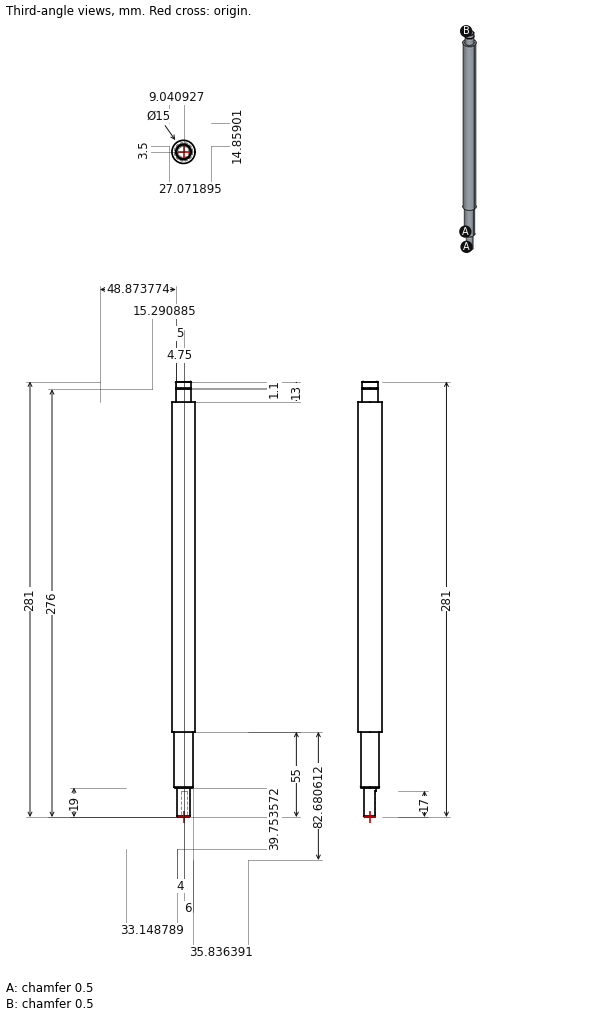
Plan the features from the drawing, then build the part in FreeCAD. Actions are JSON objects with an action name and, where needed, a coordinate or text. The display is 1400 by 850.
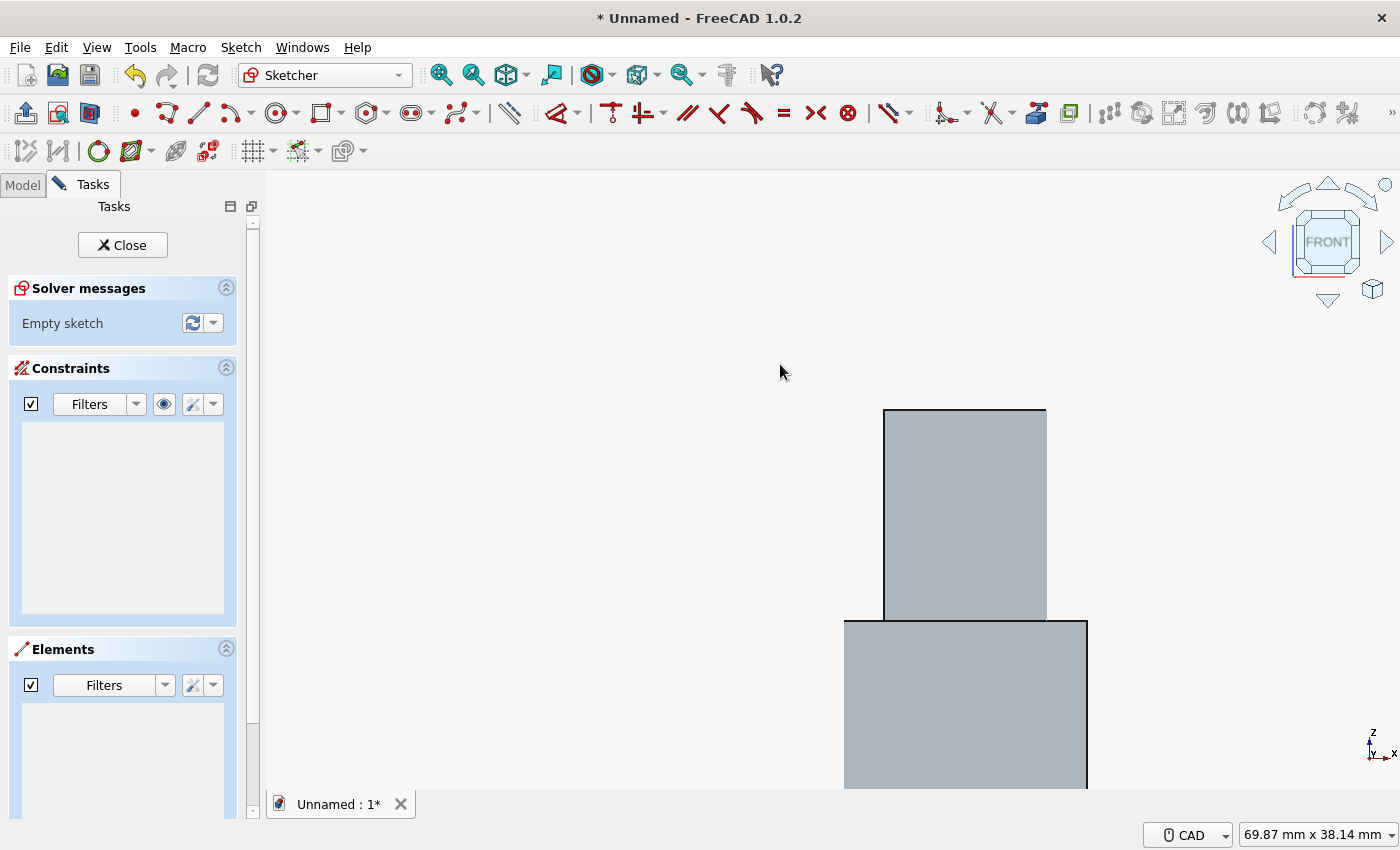
{"action": "scroll", "coordinate": [764, 484], "scroll_direction": "up", "scroll_amount": 5}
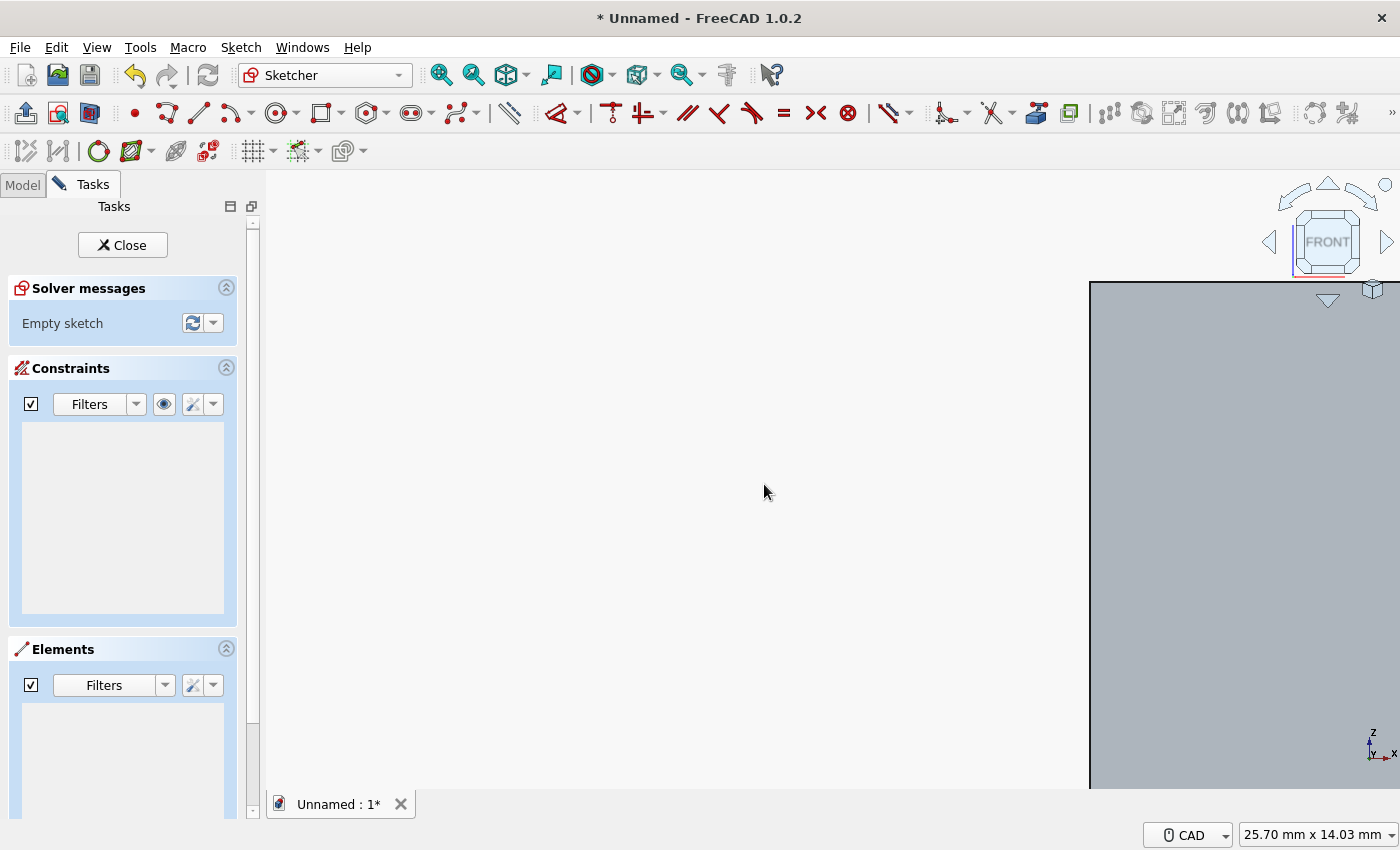
{"action": "left_click", "coordinate": [322, 114]}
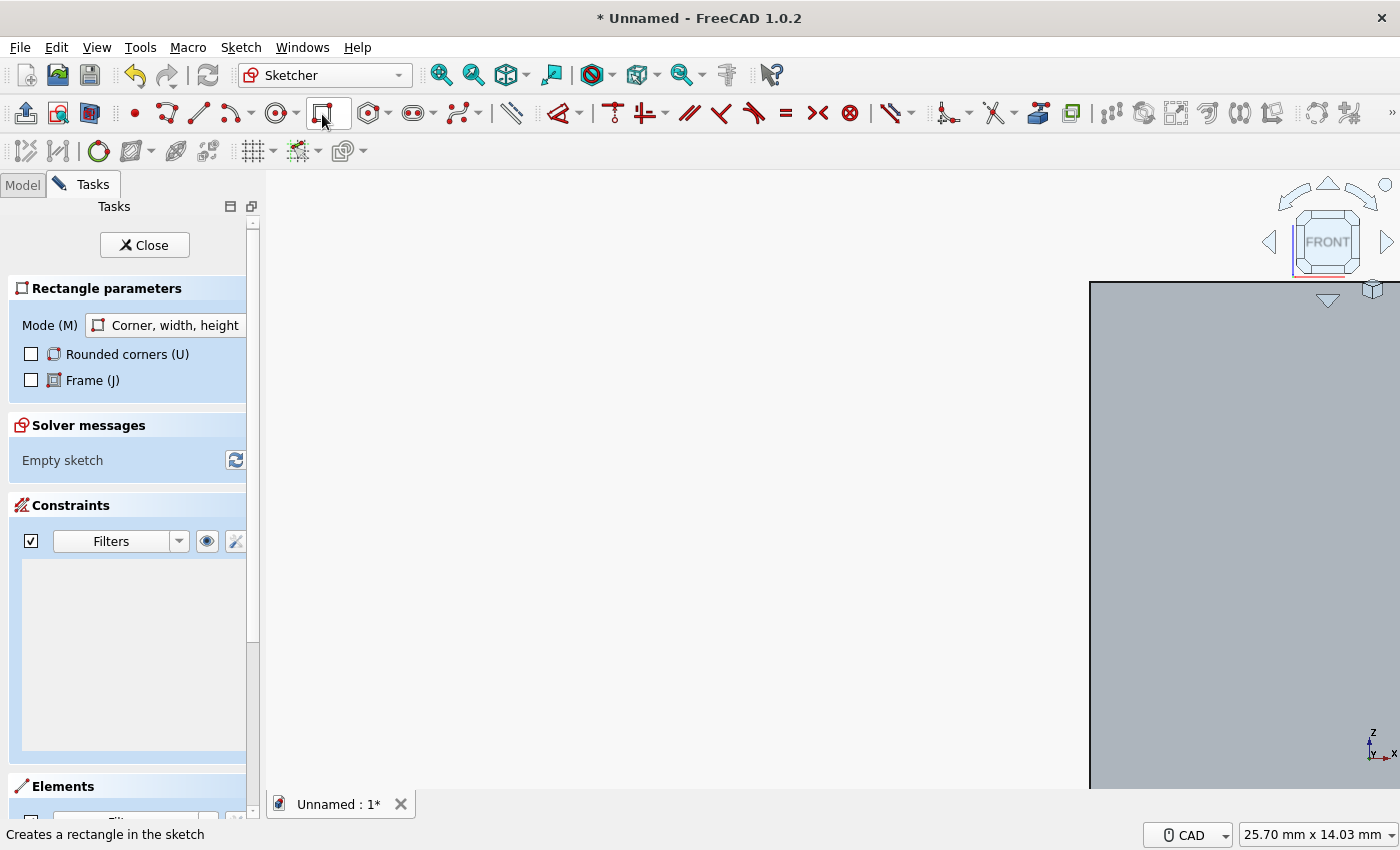
{"action": "left_click", "coordinate": [426, 454]}
{"action": "mouse_move", "coordinate": [1101, 503]}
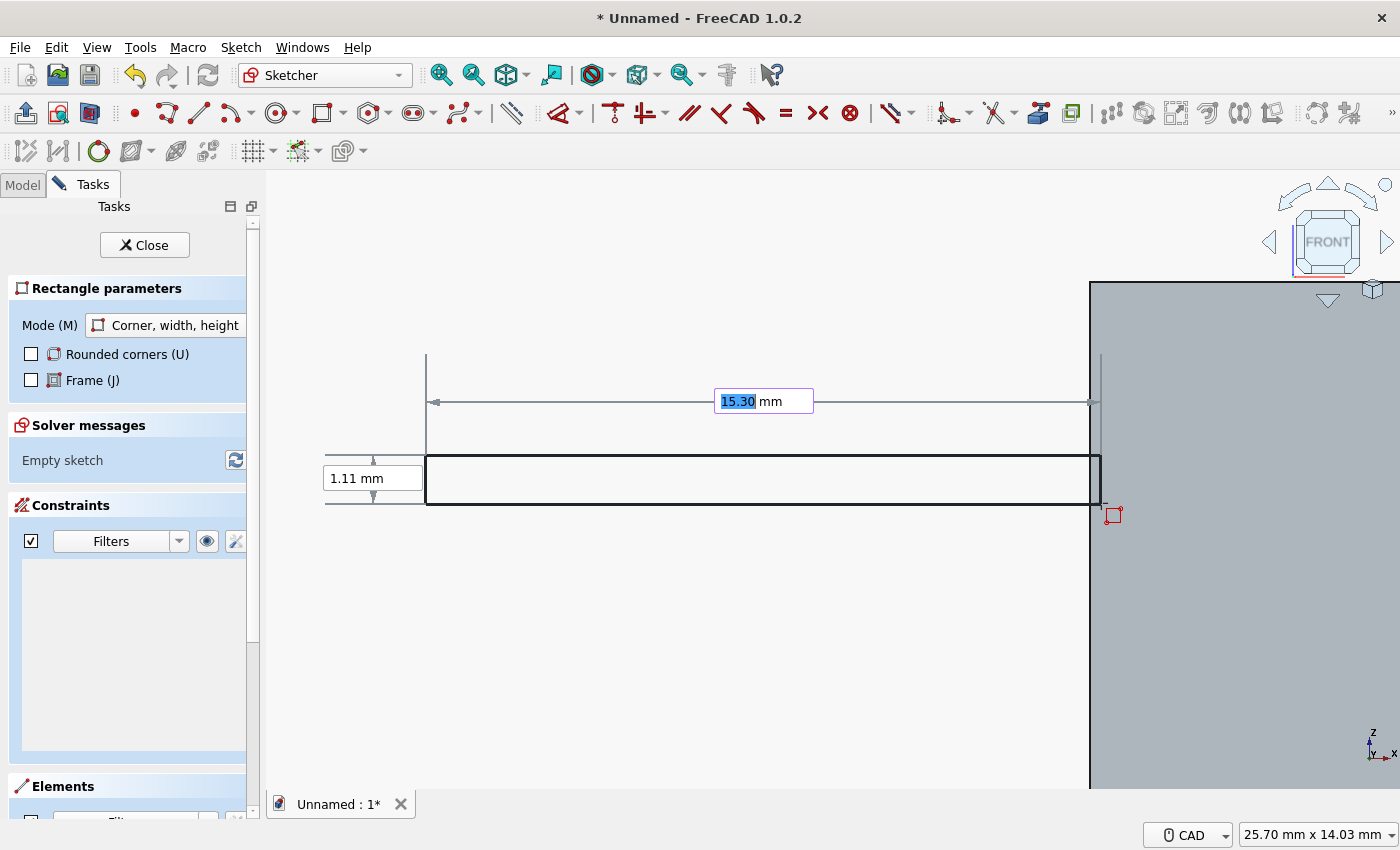
{"action": "type", "text": "15.290885"}
{"action": "key", "text": "Tab"}
{"action": "type", "text": "1.1"}
{"action": "key", "text": "Return"}
{"action": "key", "text": "Escape"}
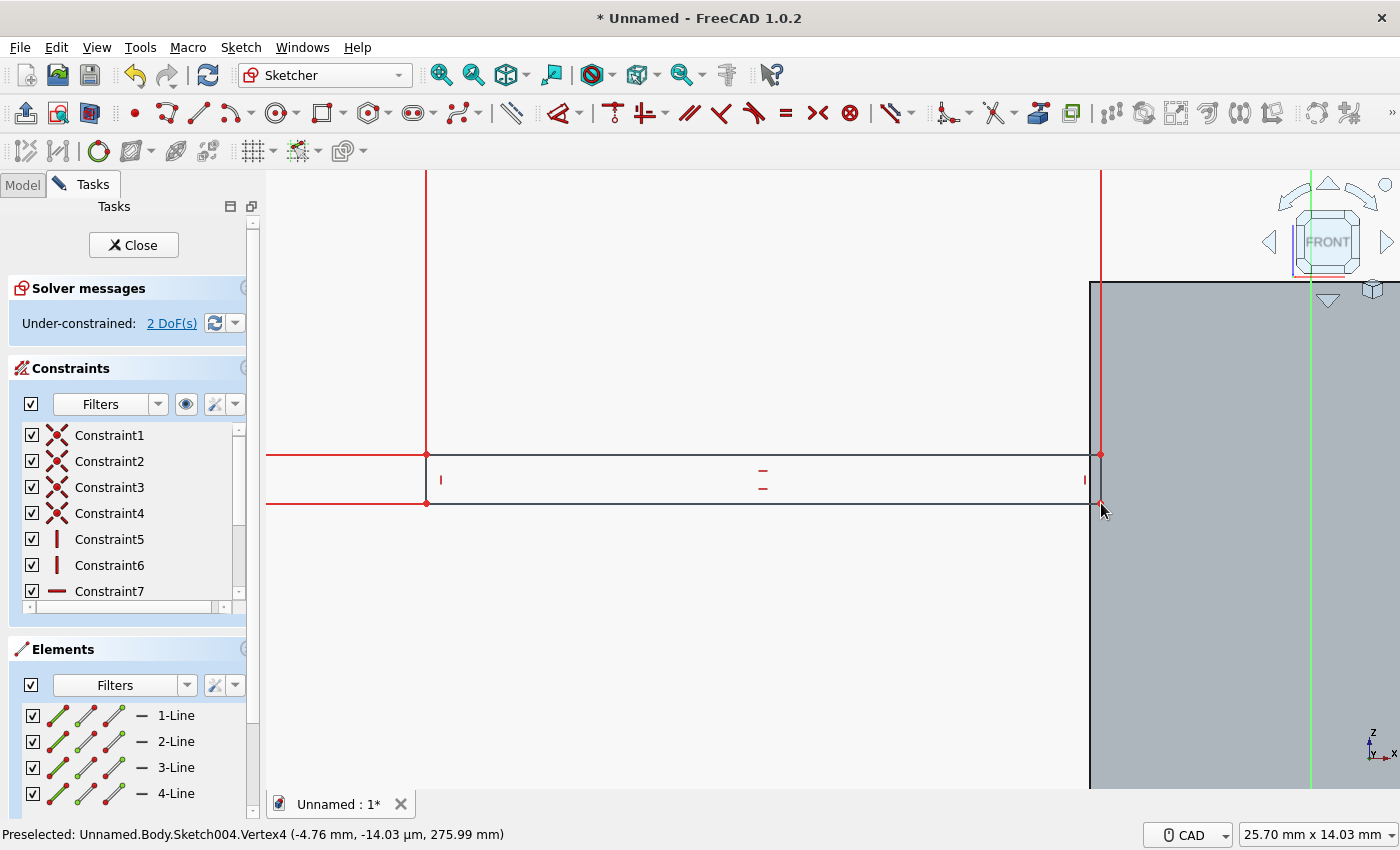
{"action": "left_click", "coordinate": [558, 114]}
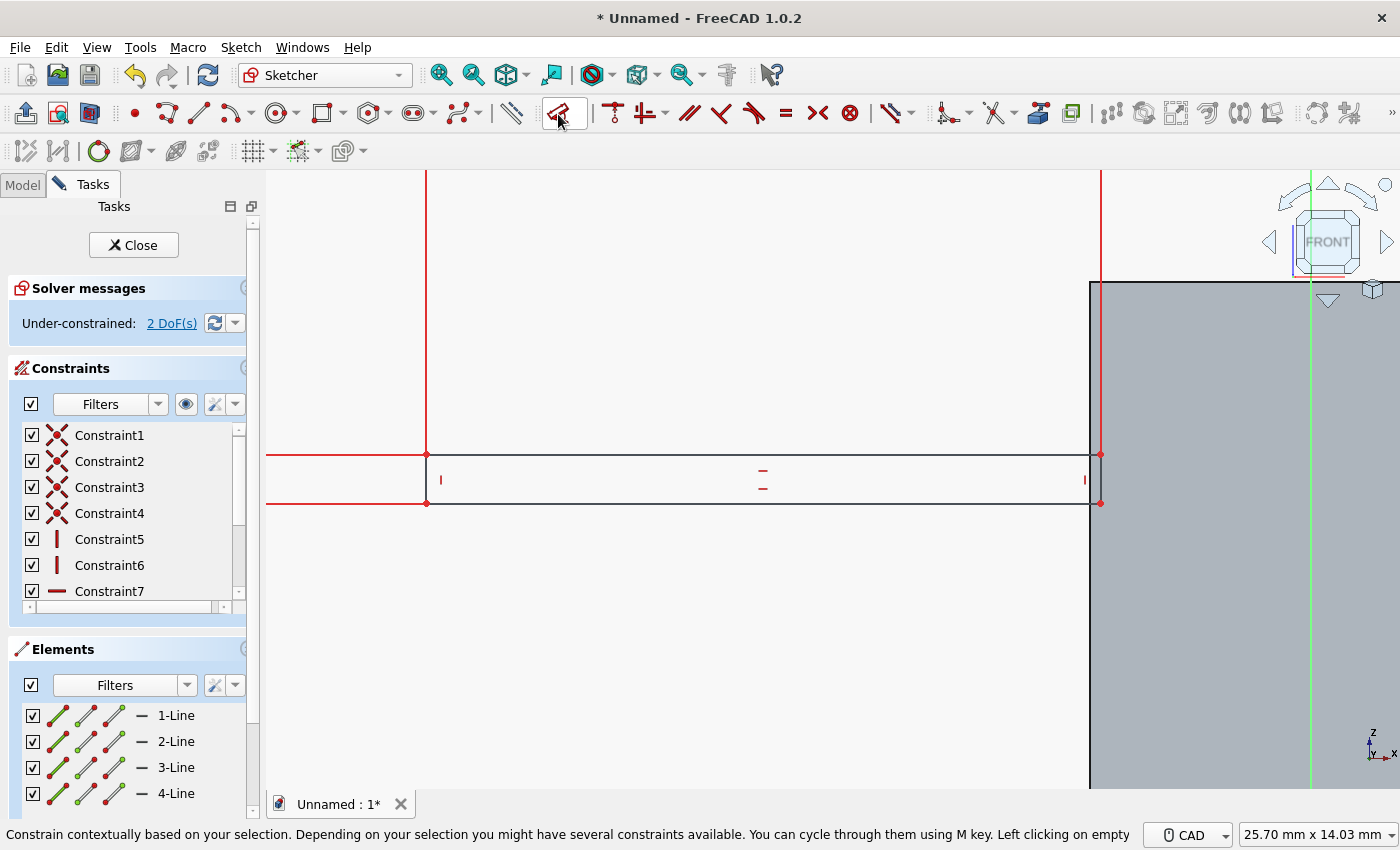
{"action": "left_click", "coordinate": [426, 504]}
{"action": "left_click", "coordinate": [392, 632]}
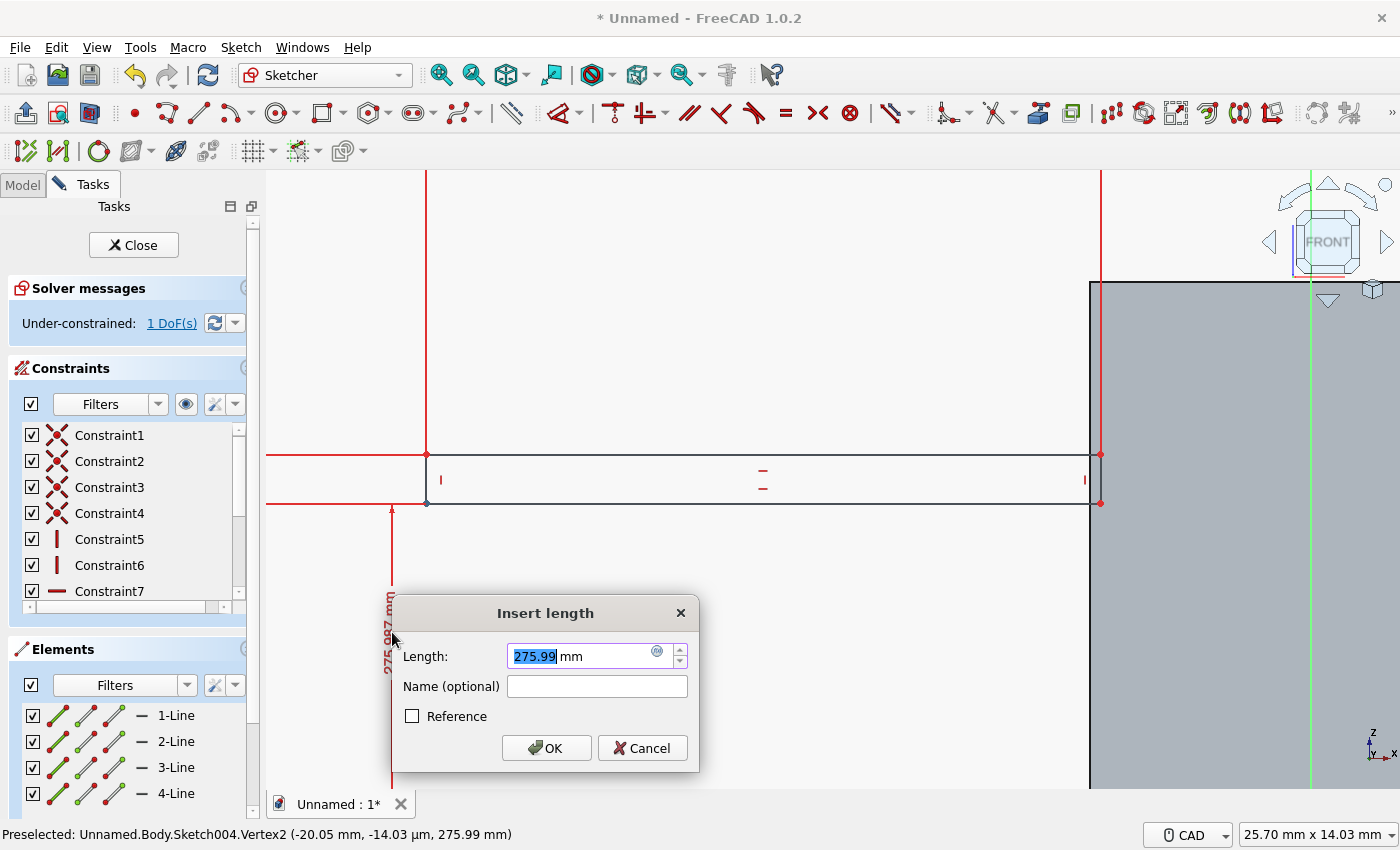
{"action": "type", "text": "276"}
{"action": "key", "text": "Return"}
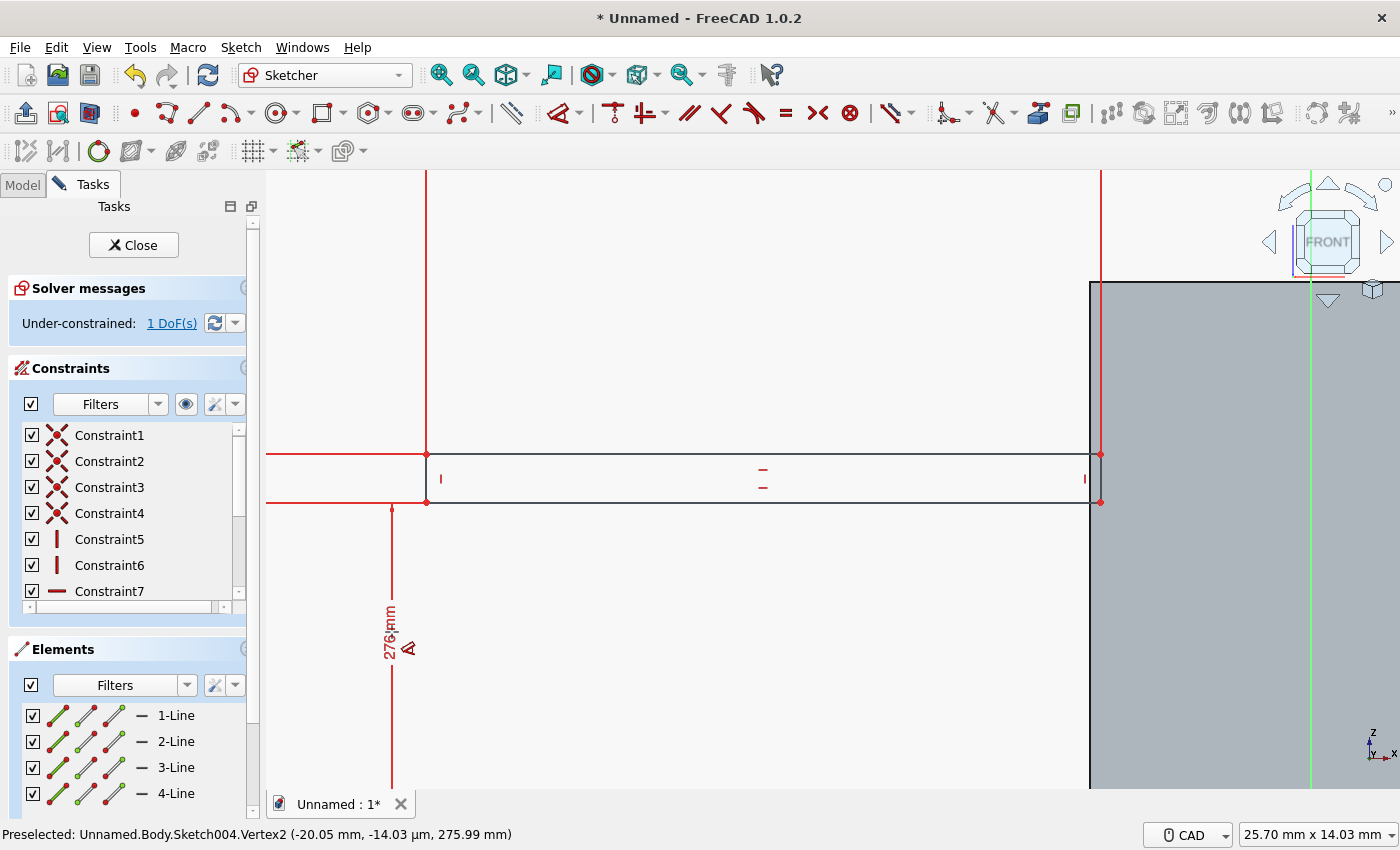
{"action": "left_click", "coordinate": [1101, 503]}
{"action": "left_click", "coordinate": [1168, 469]}